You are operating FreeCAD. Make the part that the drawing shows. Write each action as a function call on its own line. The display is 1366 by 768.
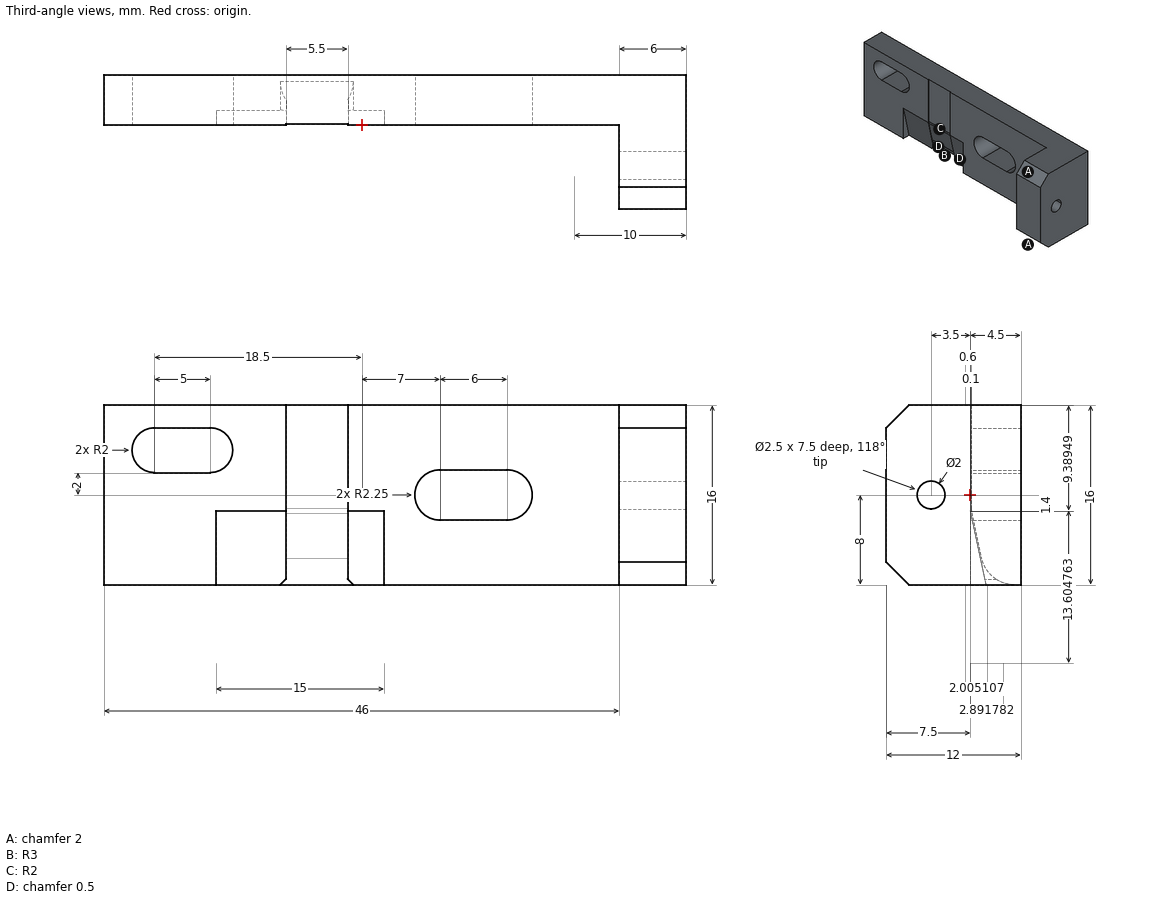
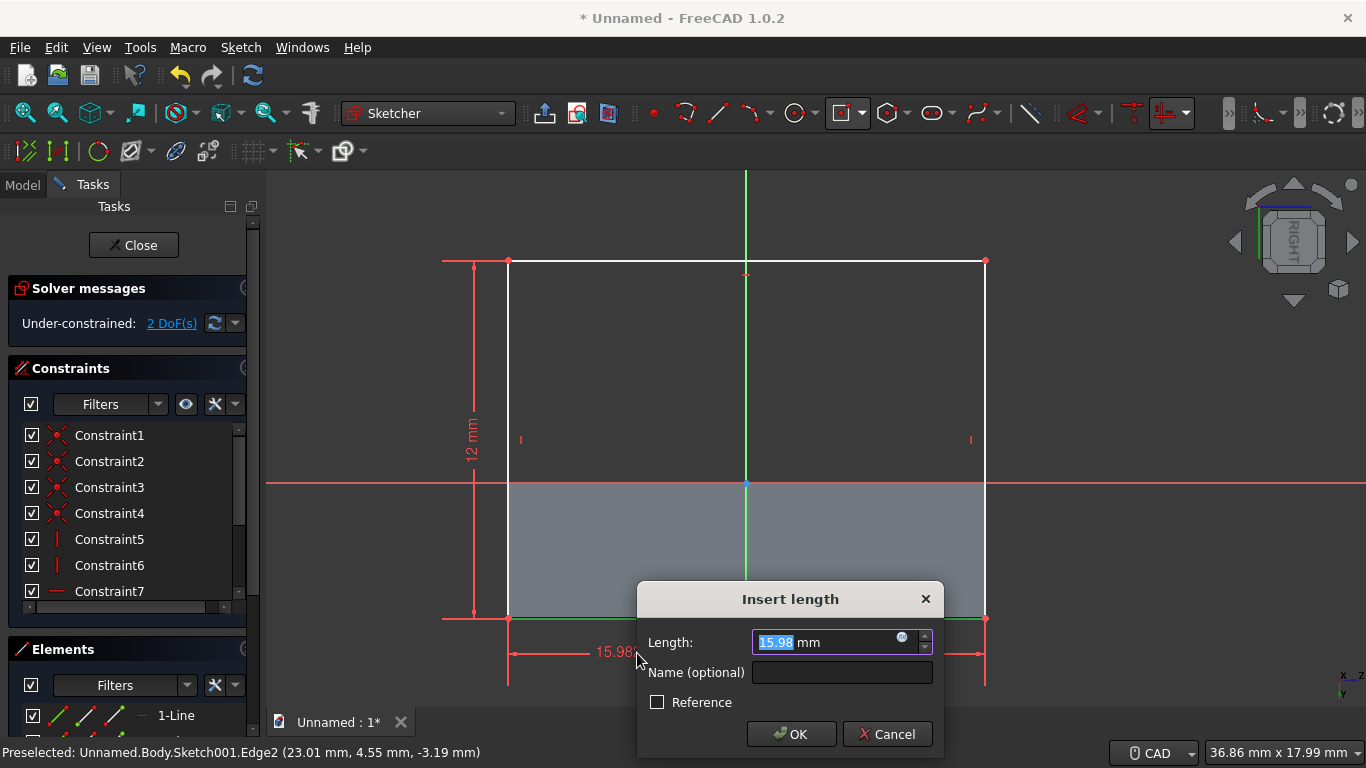
text(16)
key(Return)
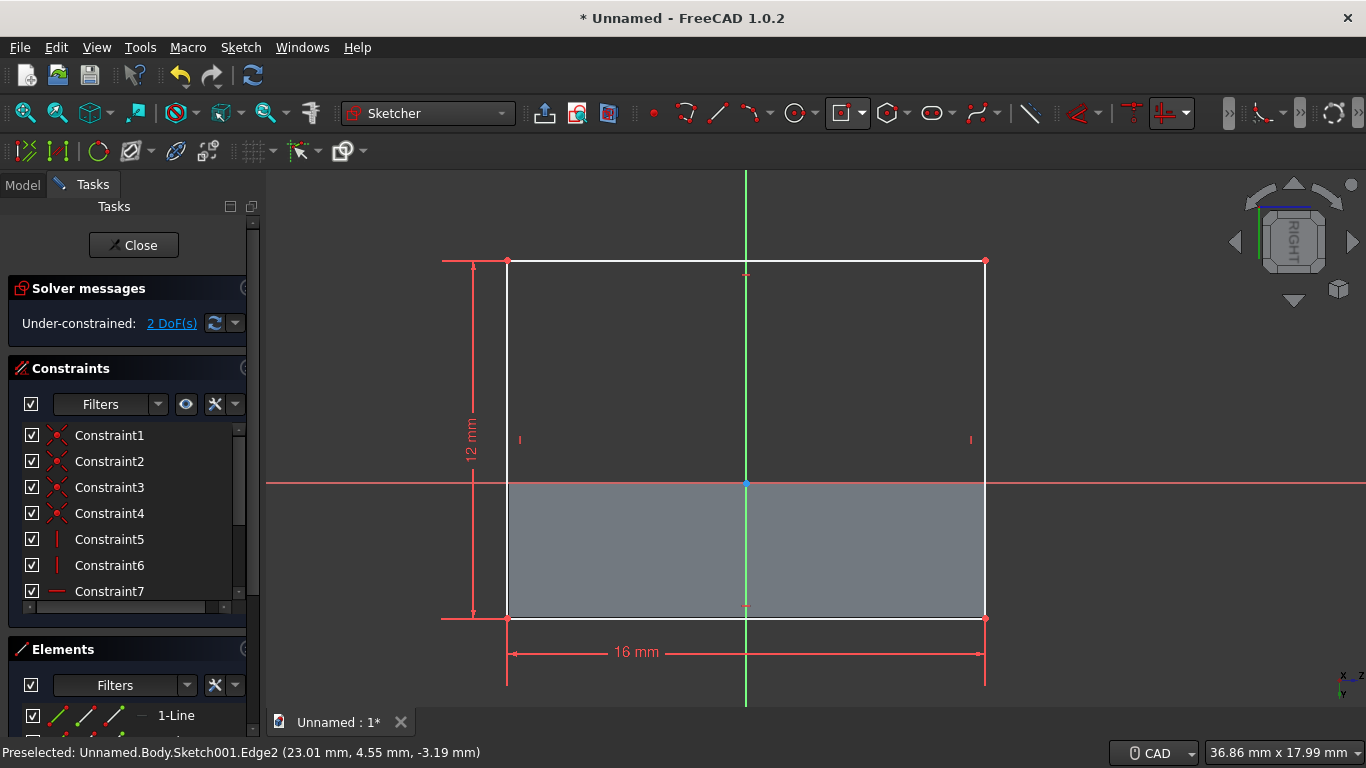
click(507, 261)
click(627, 227)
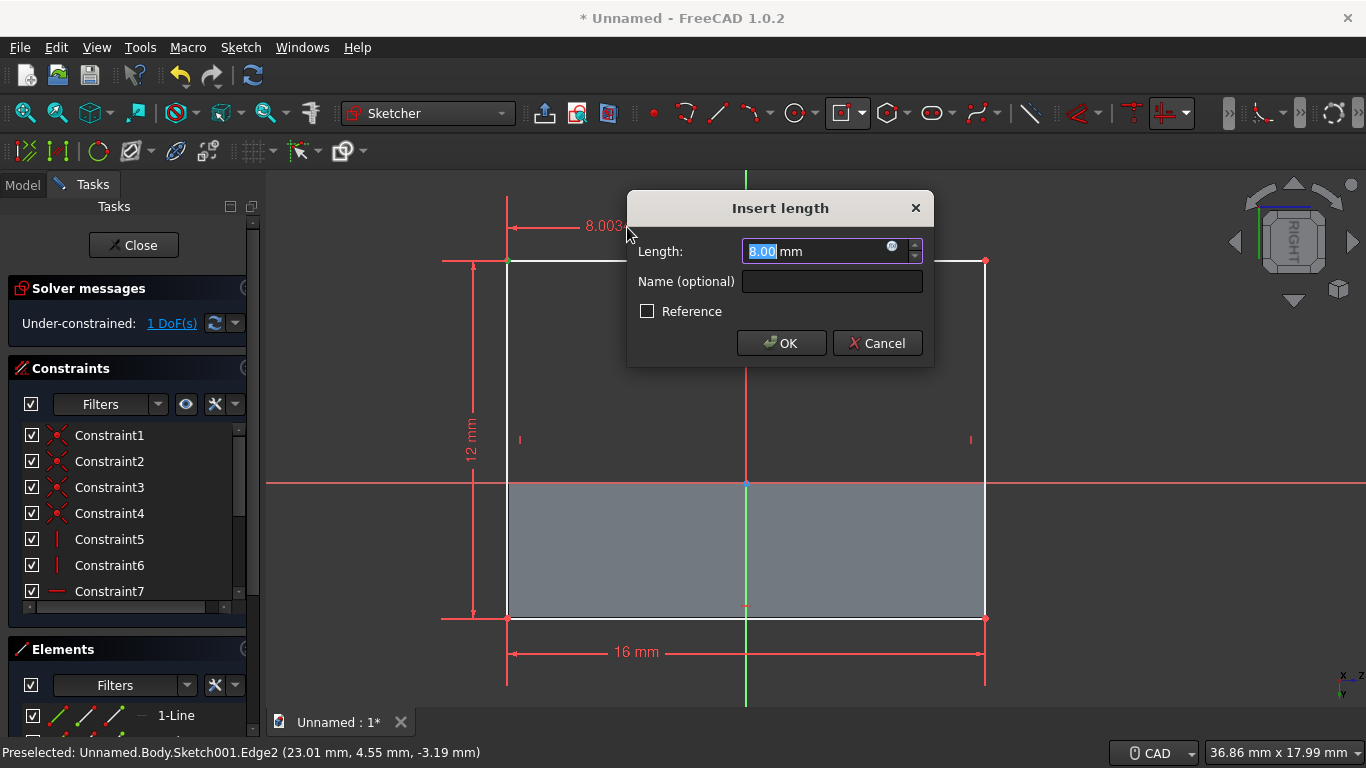
text(8)
key(Return)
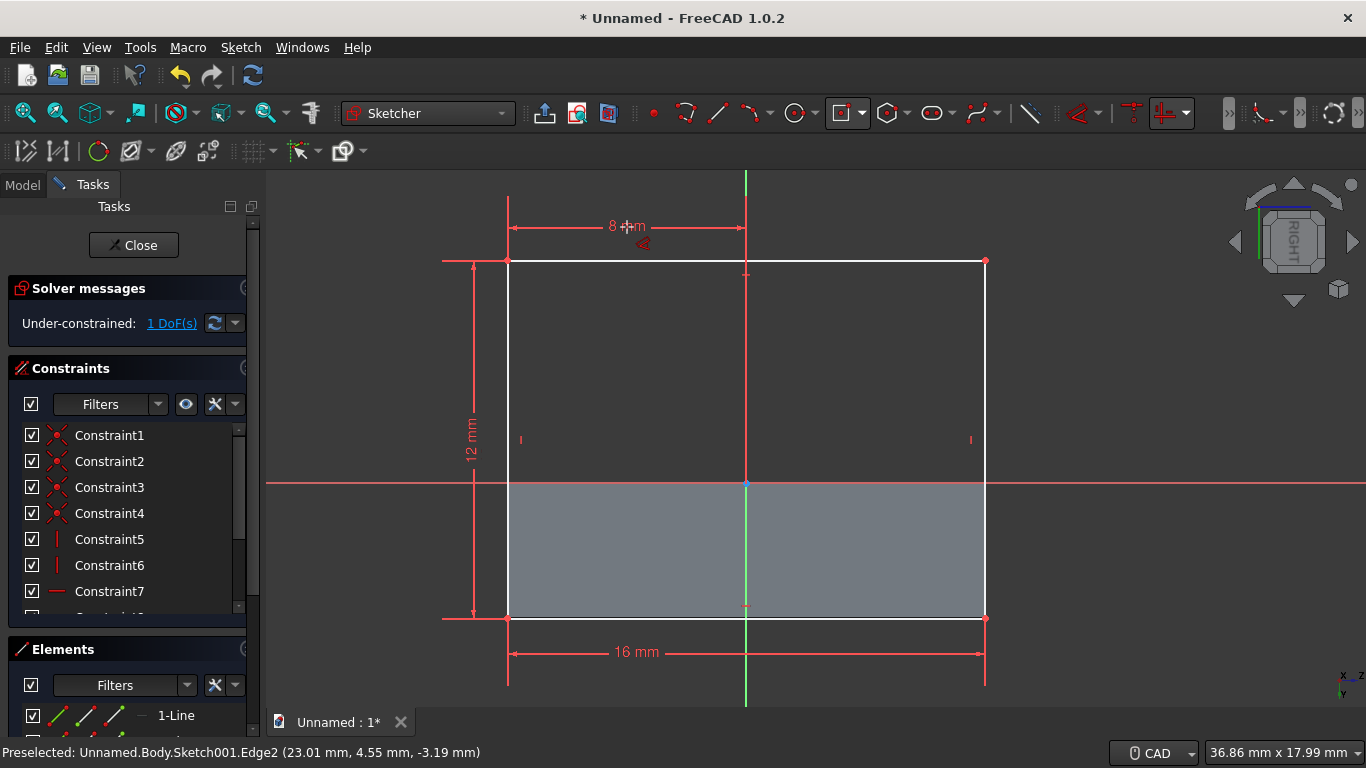
click(508, 261)
click(474, 372)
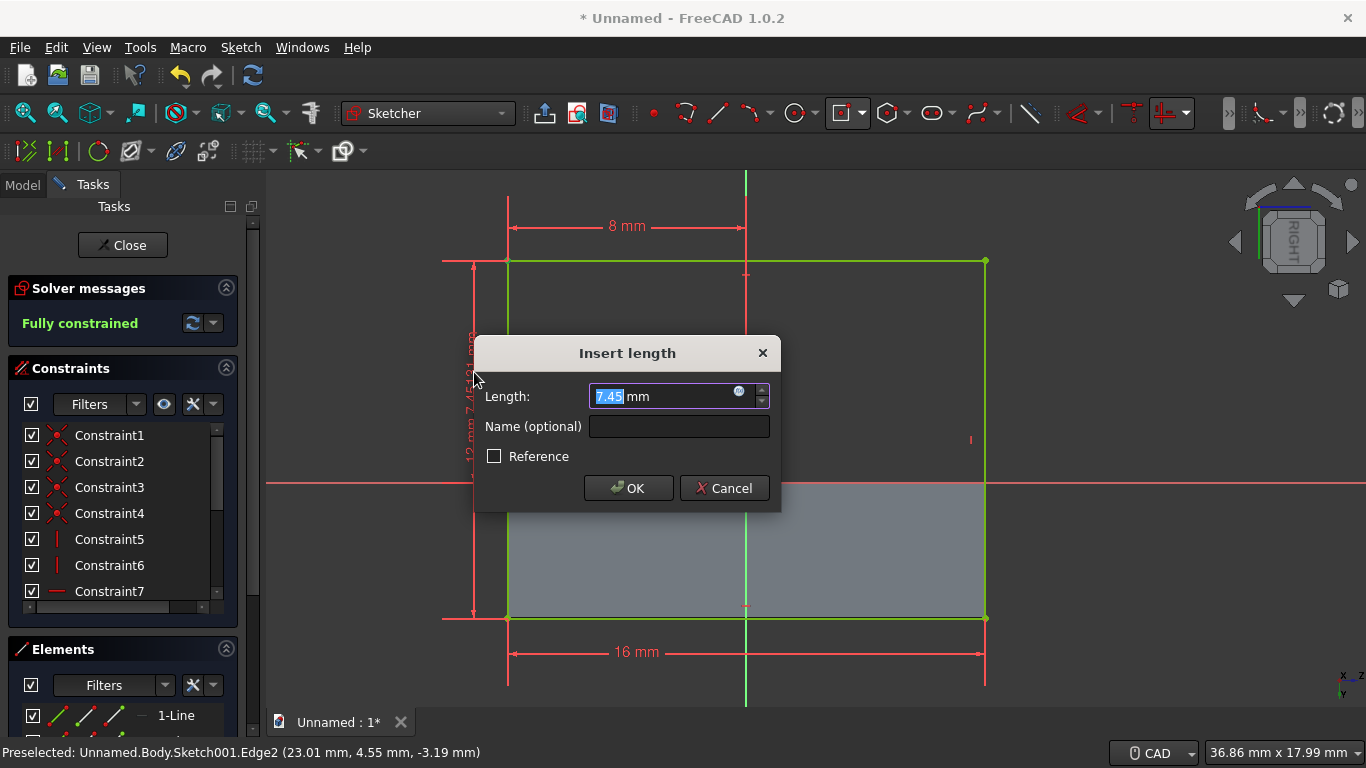
text(7.5)
key(Return)
key(Escape)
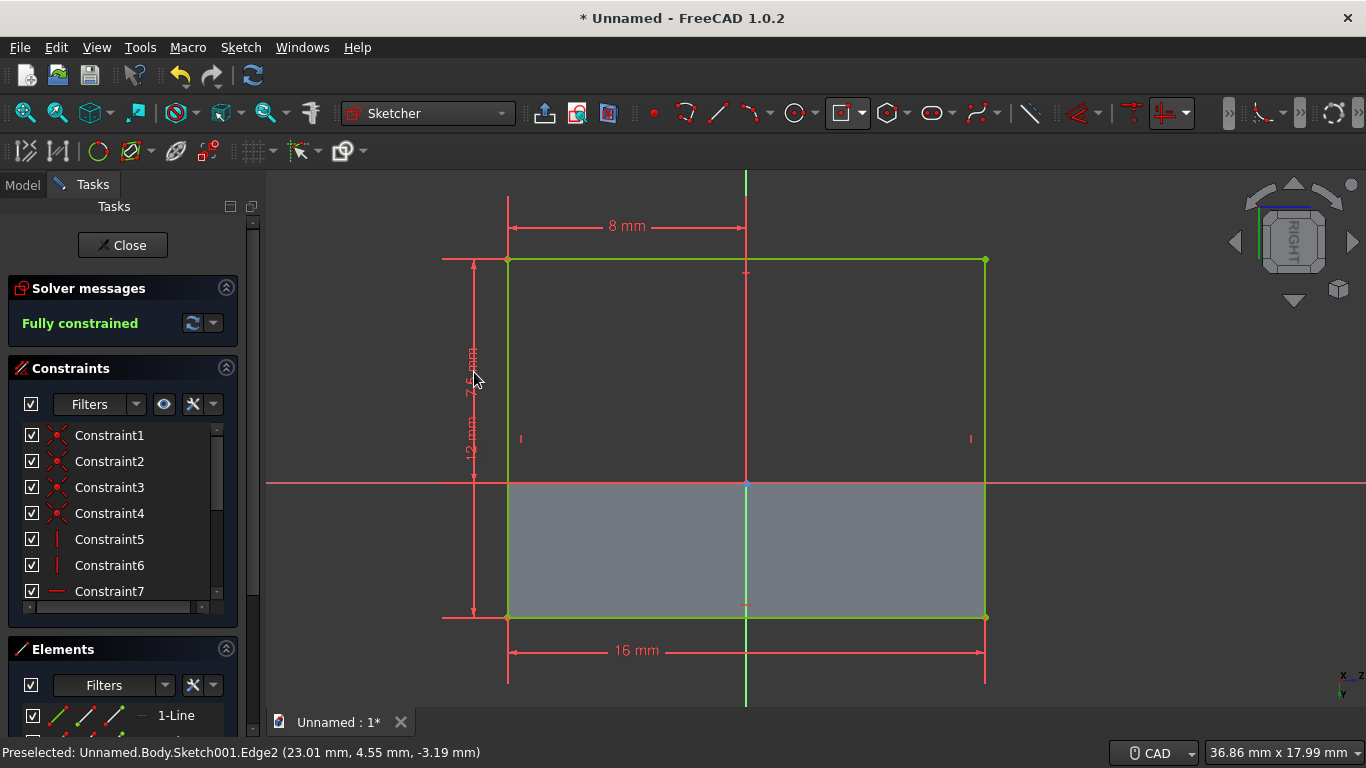
click(123, 245)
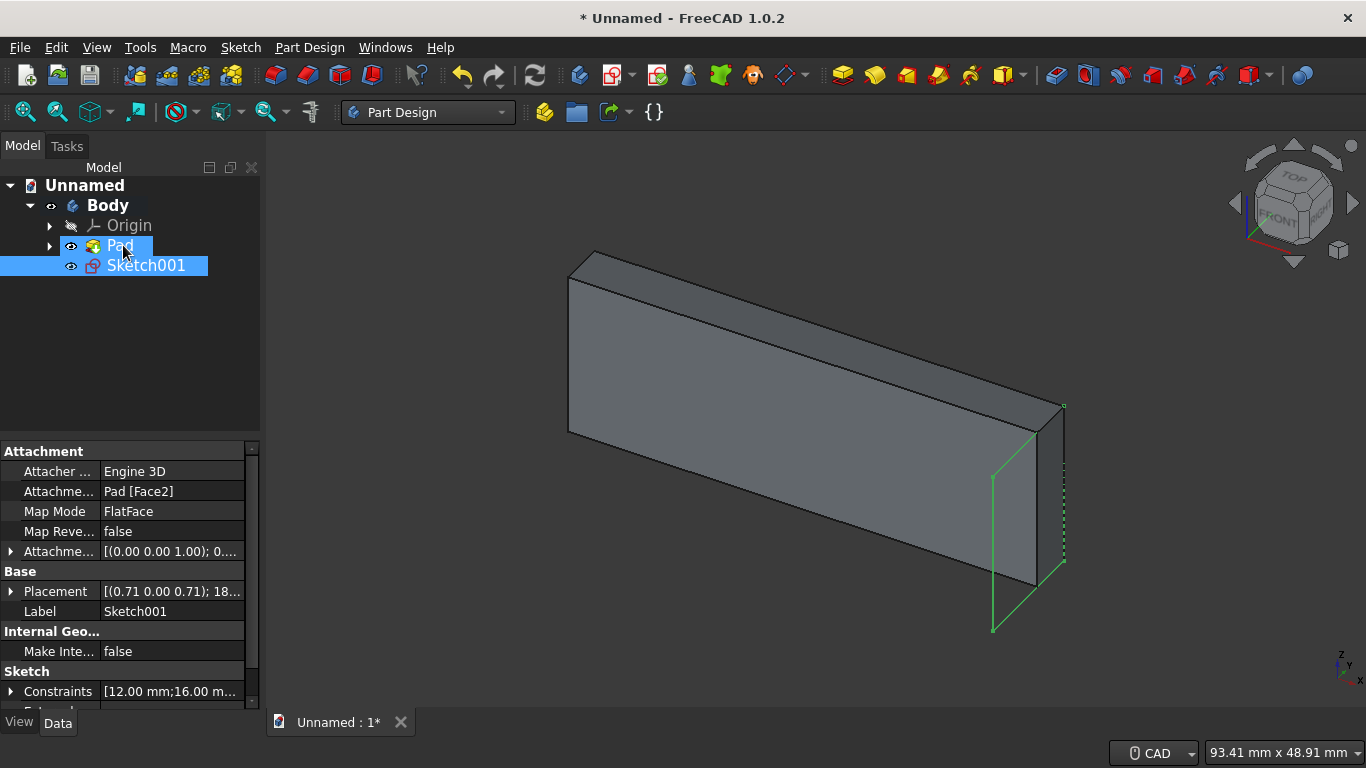
click(844, 76)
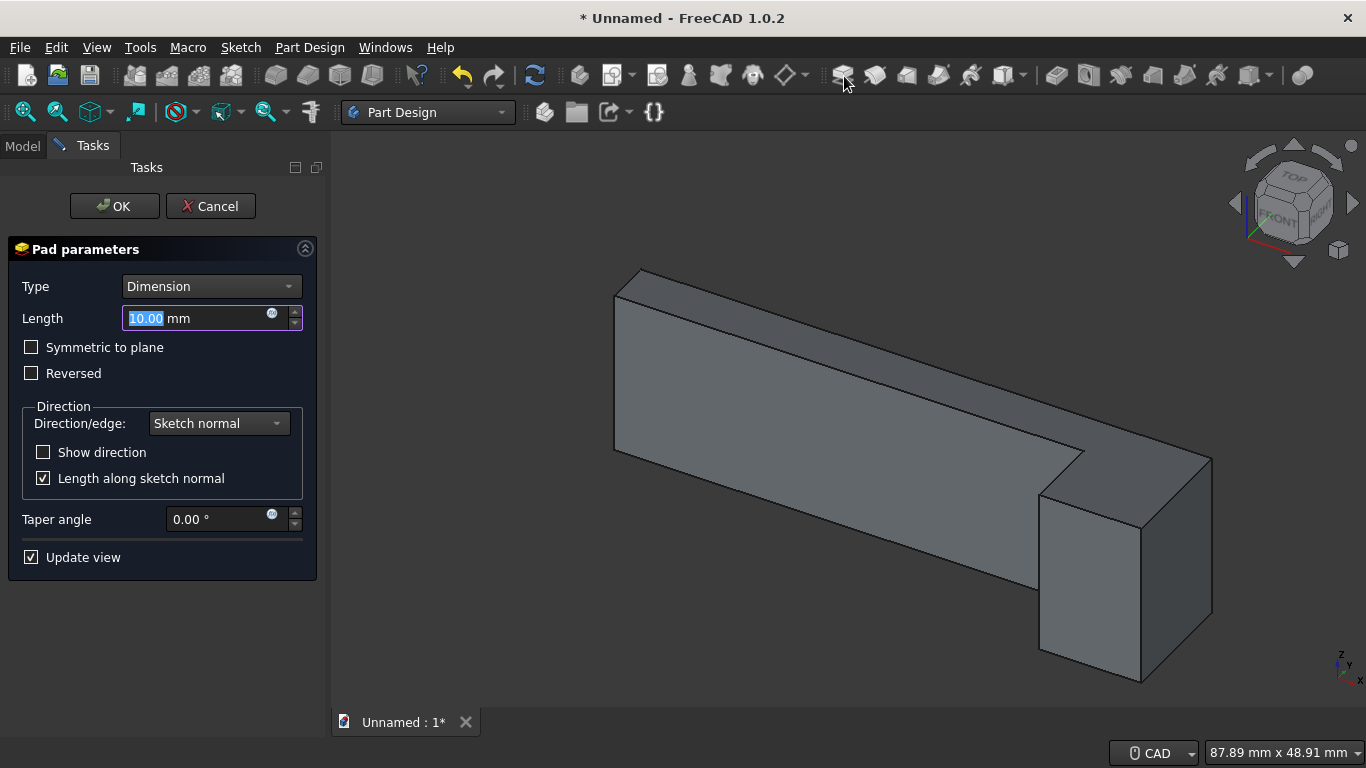
text(6)
key(Tab)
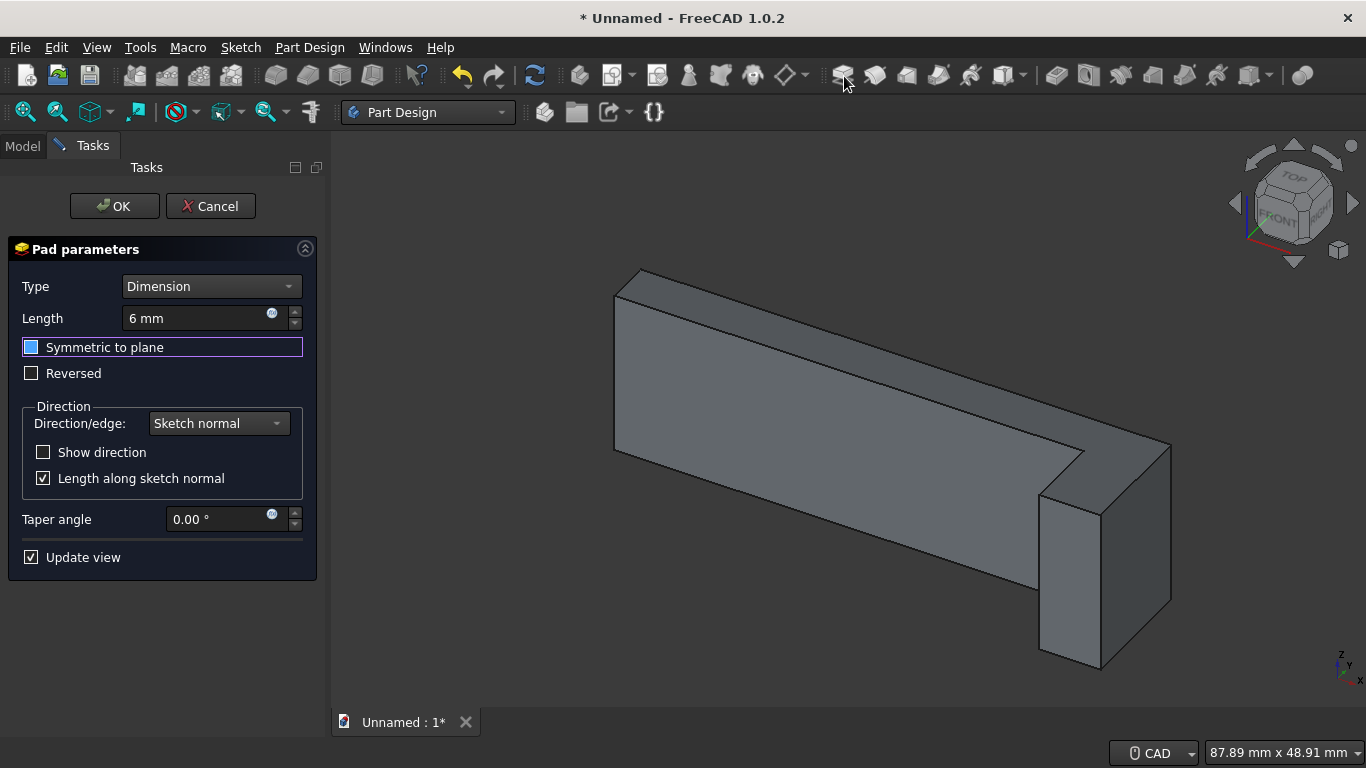
click(115, 206)